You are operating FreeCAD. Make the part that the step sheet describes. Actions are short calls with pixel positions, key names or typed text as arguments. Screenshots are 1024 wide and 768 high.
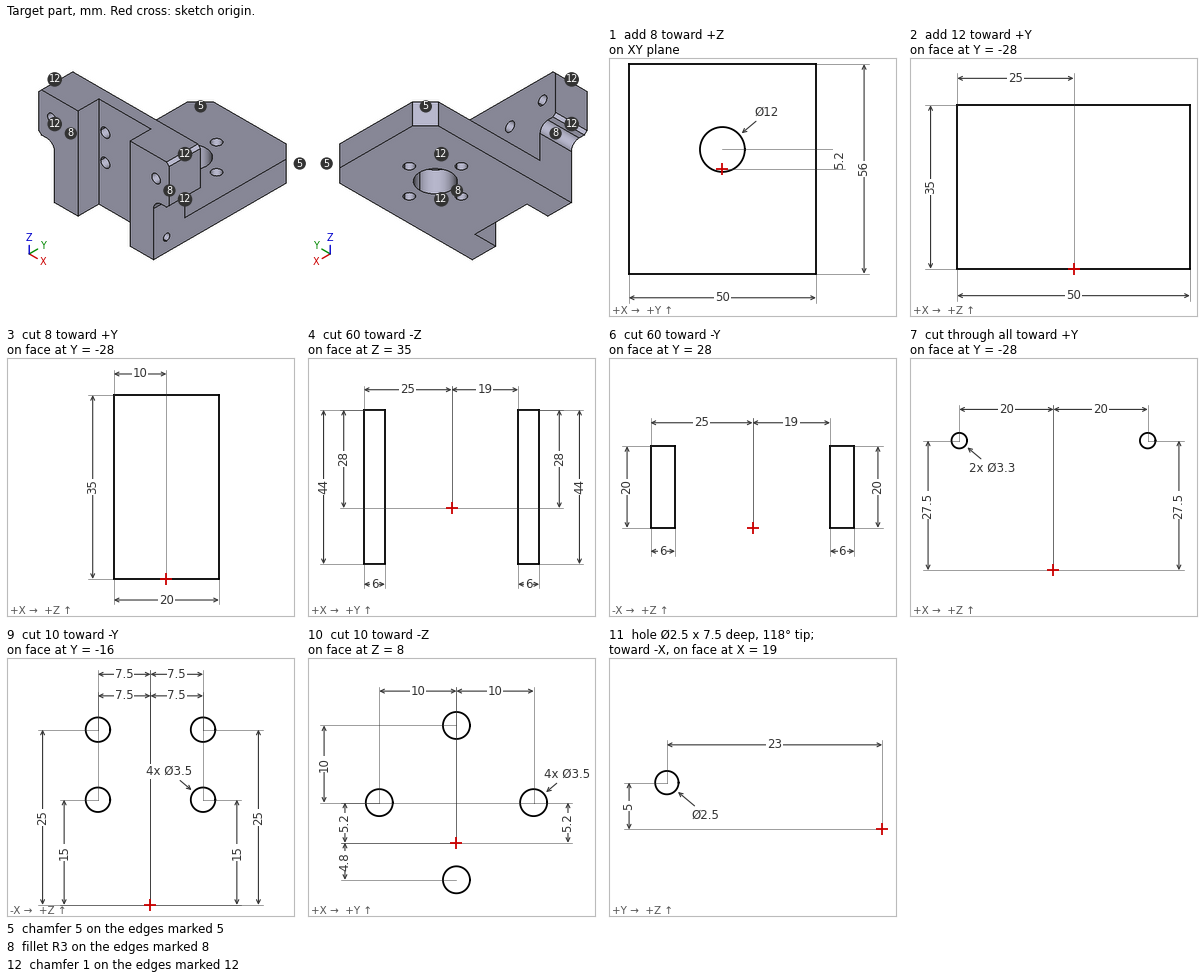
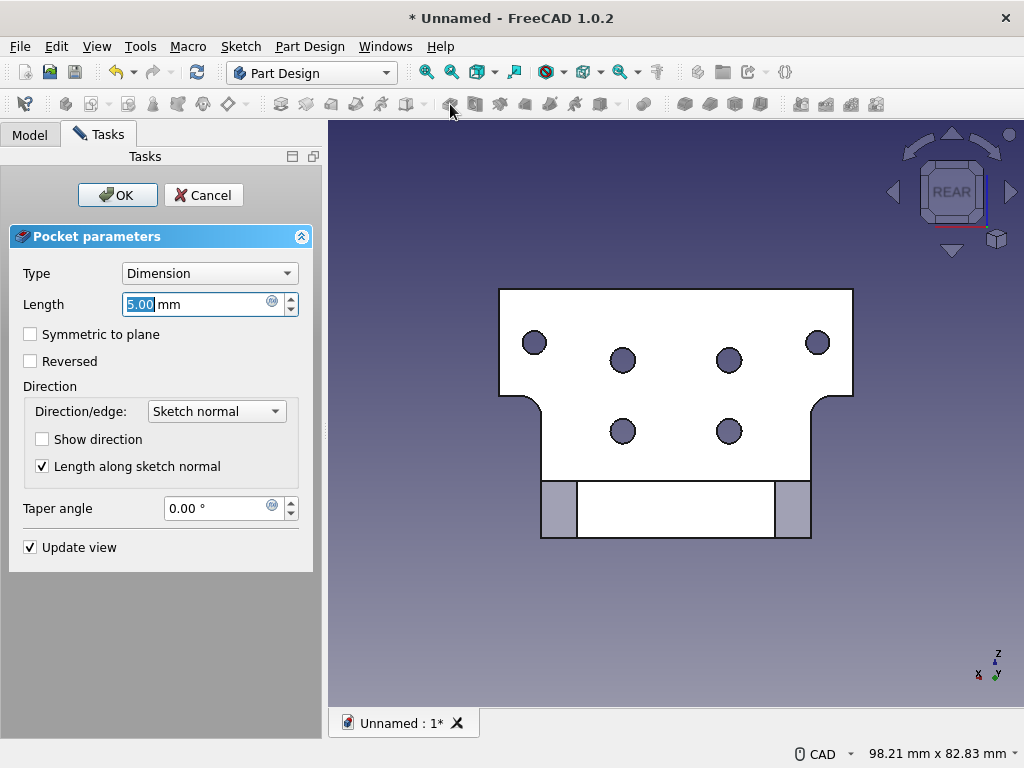
text(10)
key(Tab)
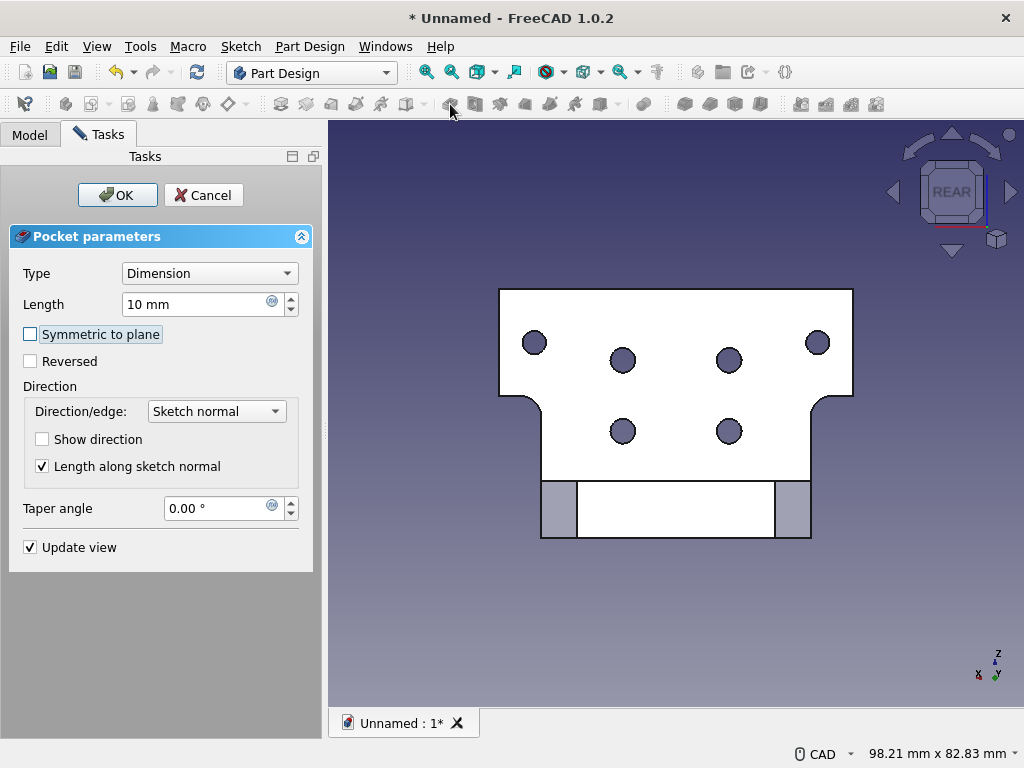
click(118, 195)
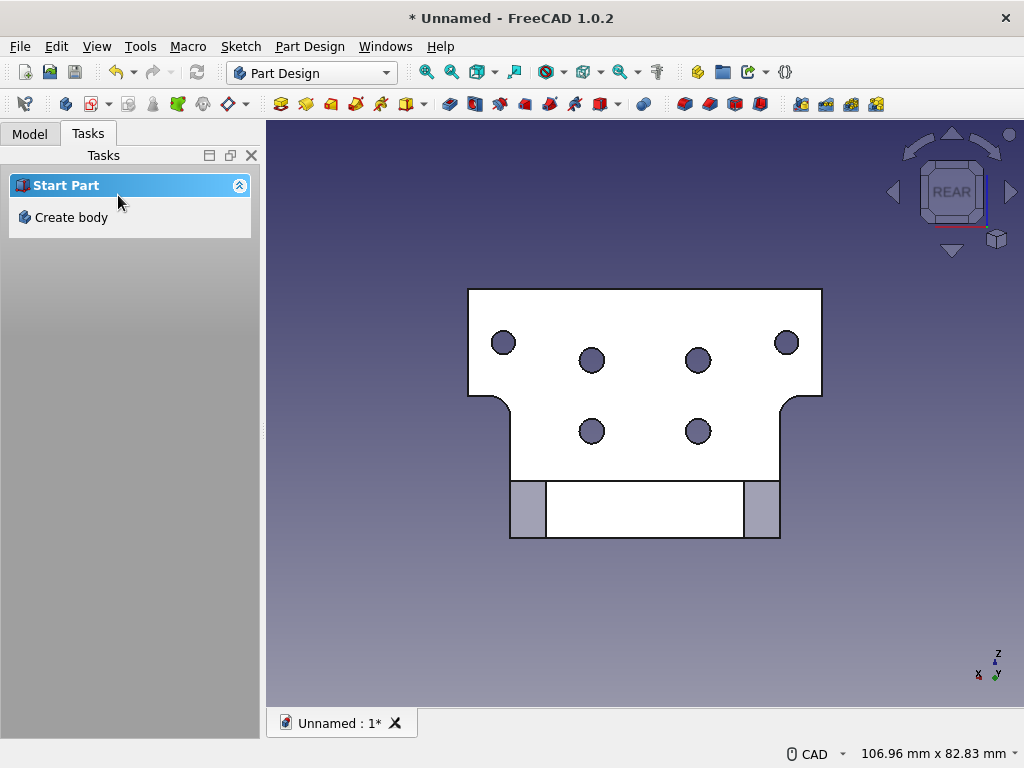
key(0)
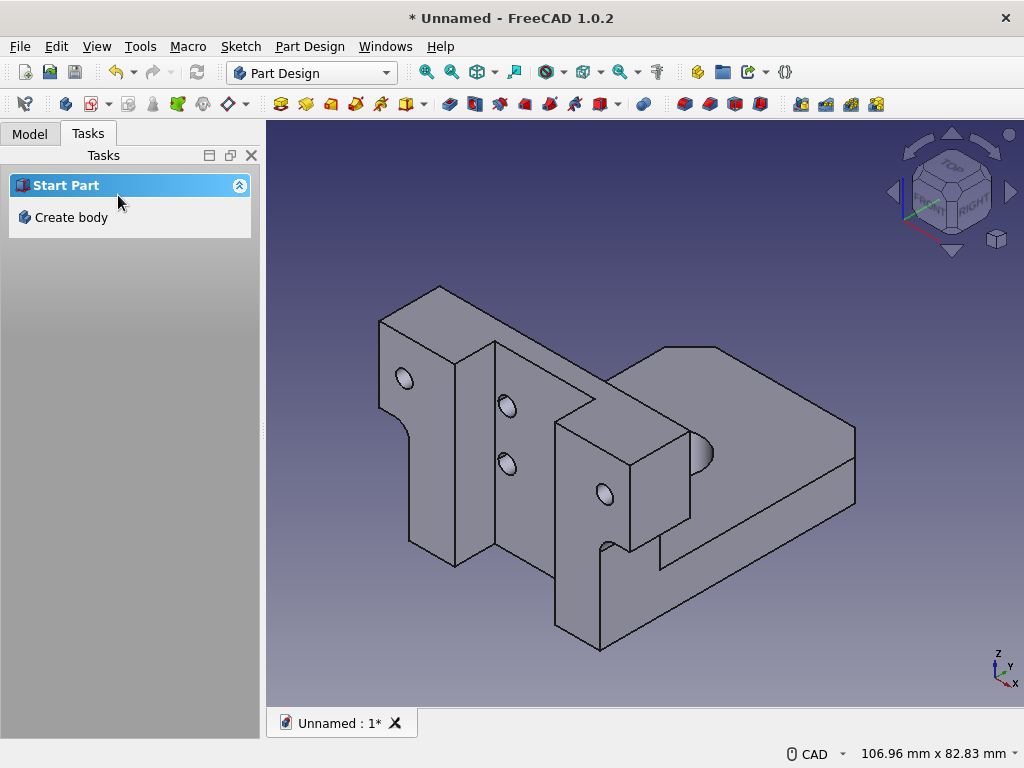
click(711, 398)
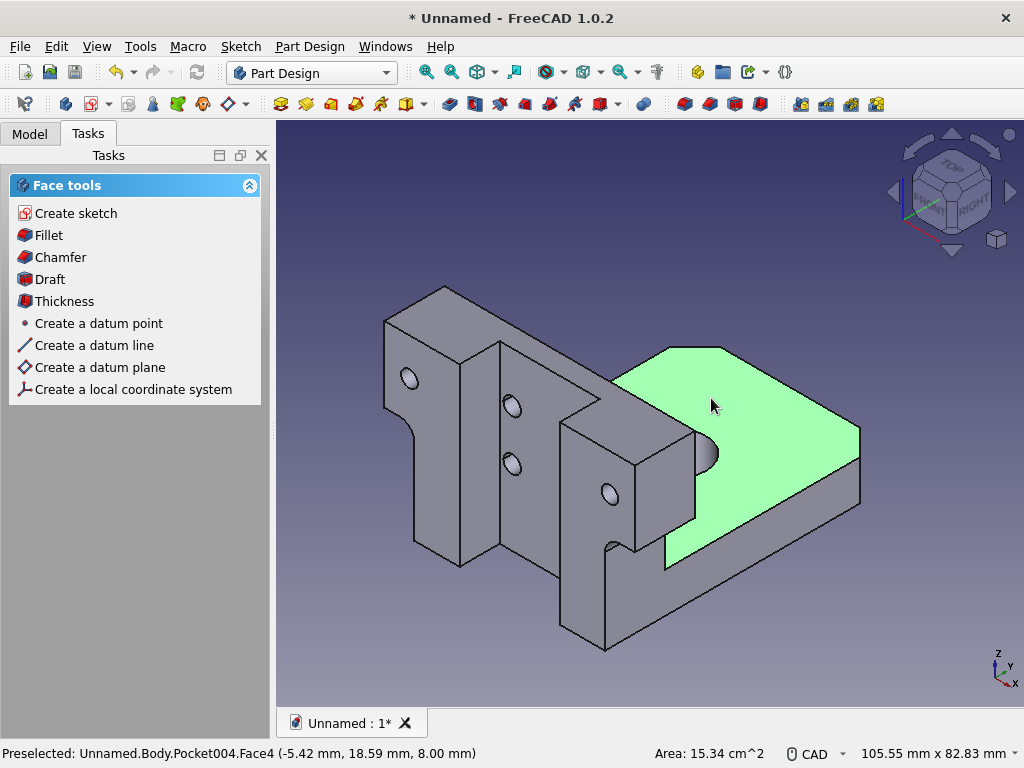
click(90, 104)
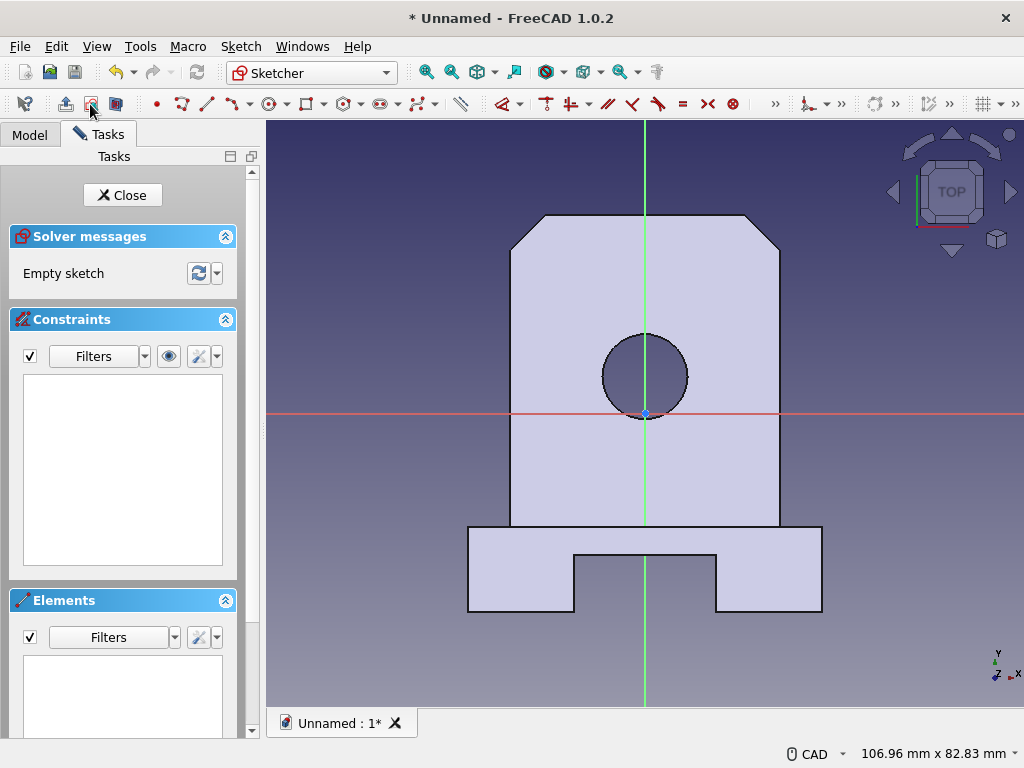
scroll(701, 347, up, 4)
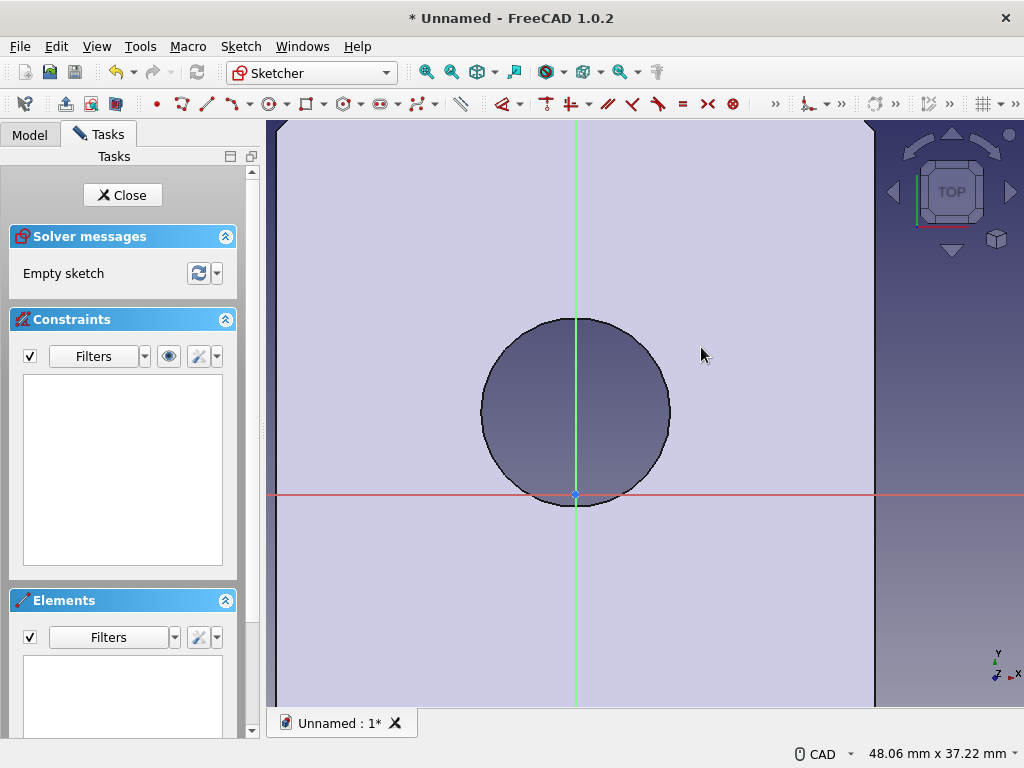
click(268, 104)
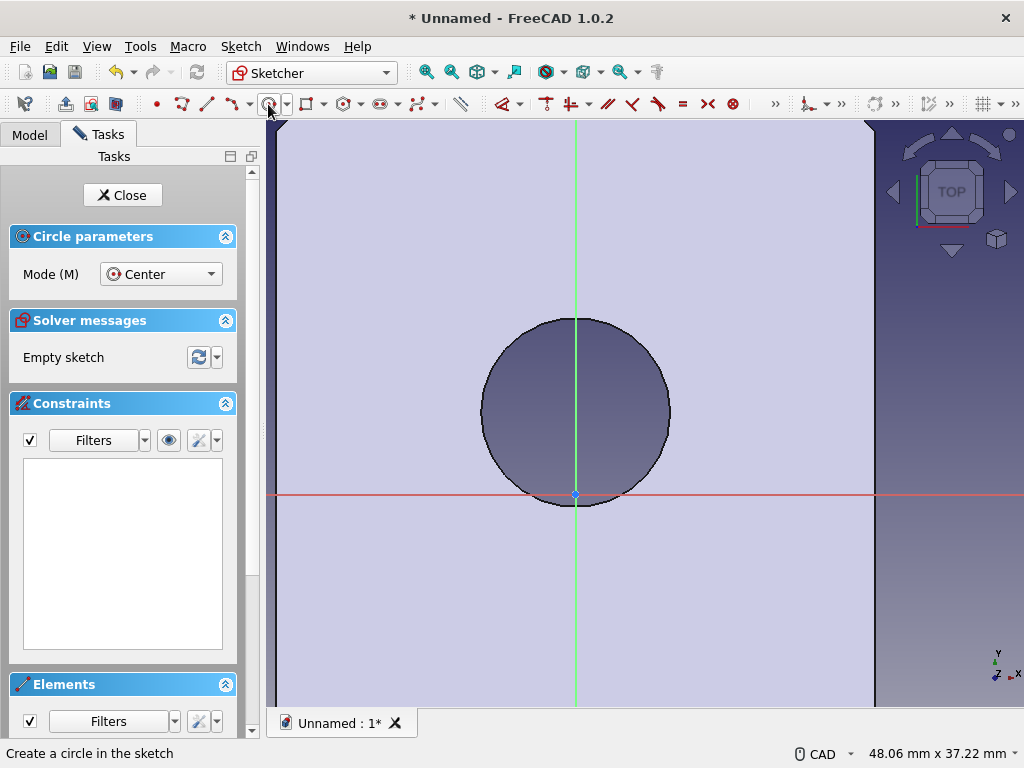
click(733, 413)
move(753, 393)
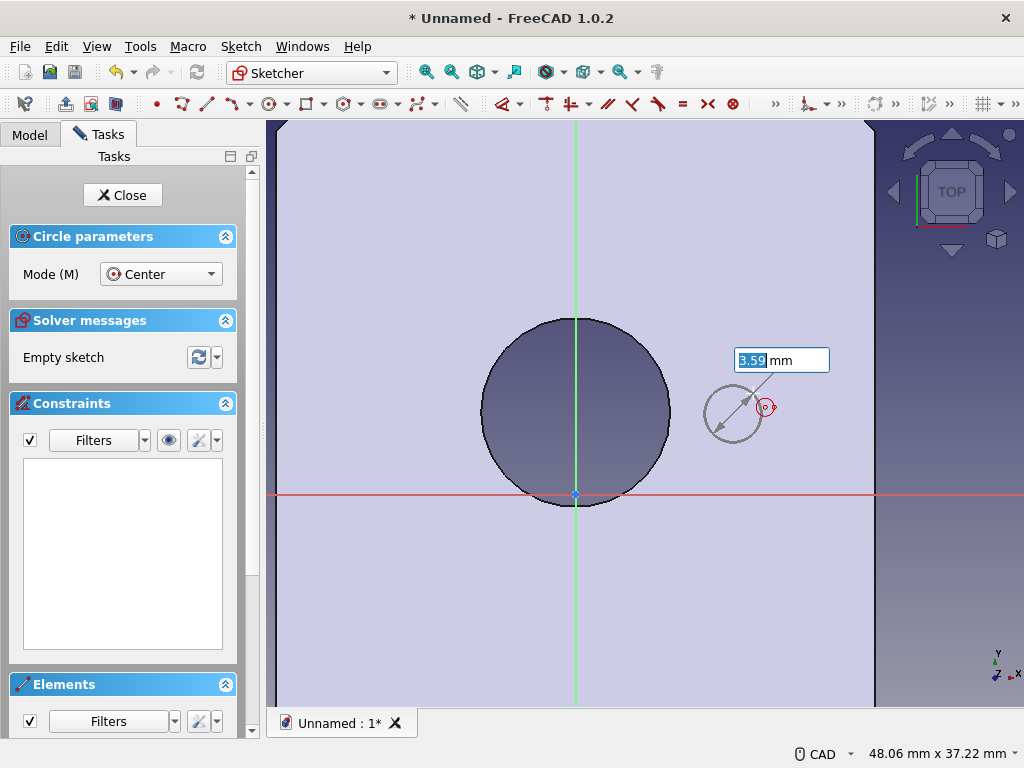
text(3.5)
key(Return)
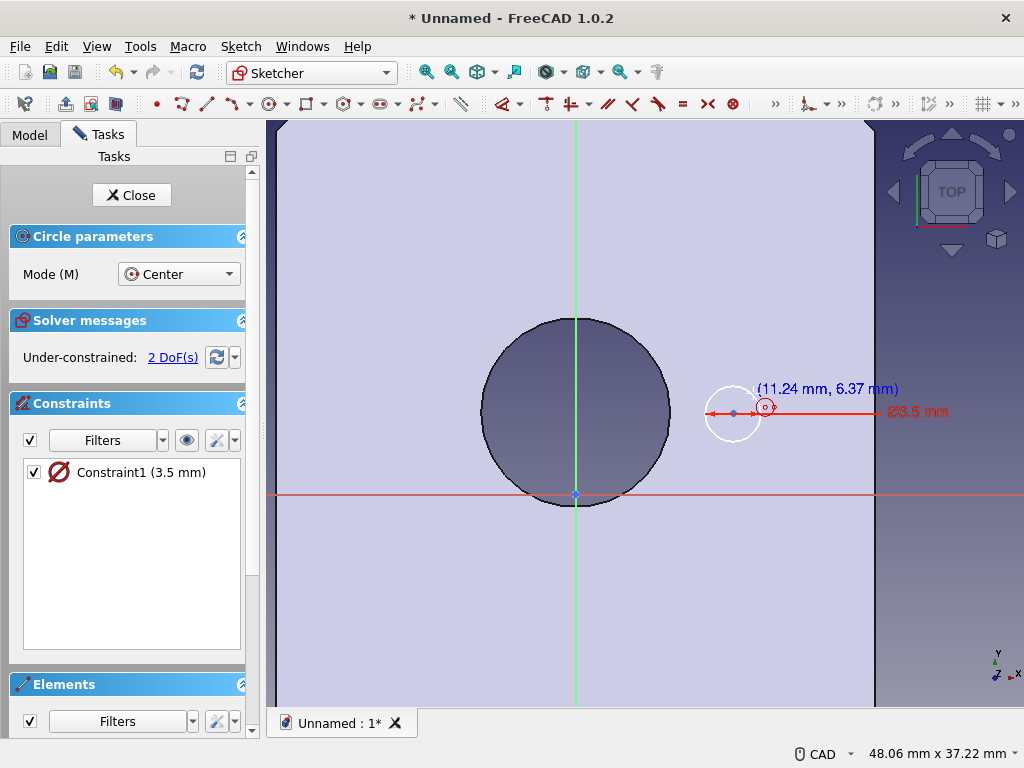
click(576, 255)
move(595, 235)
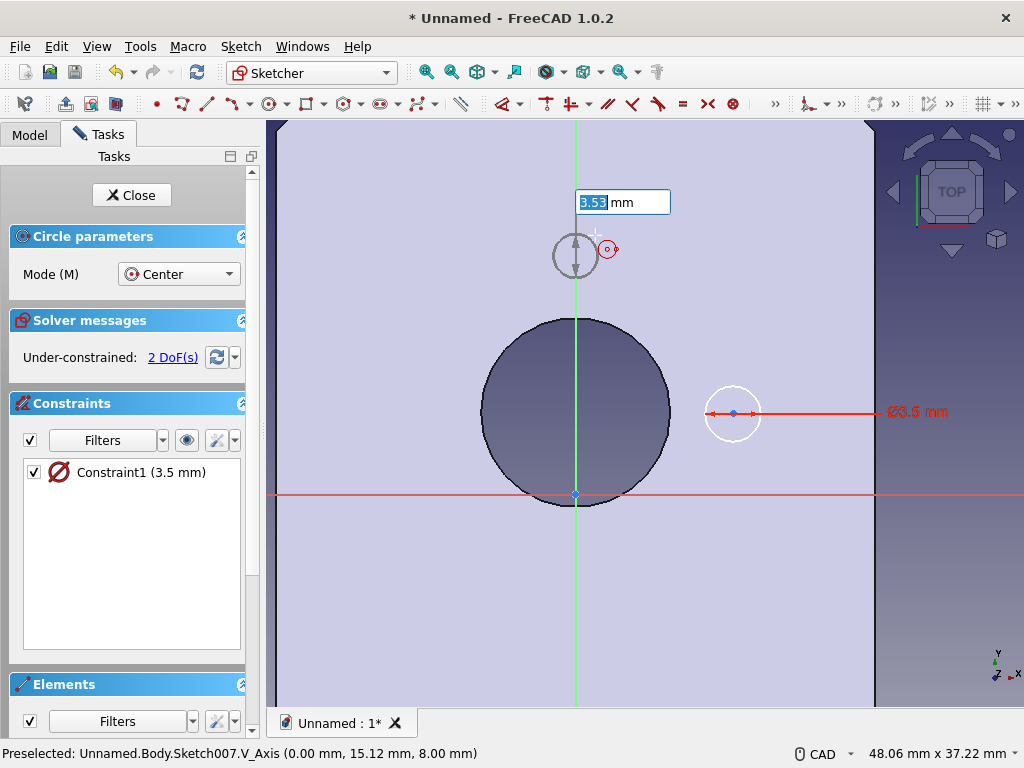
text(3.5)
key(Return)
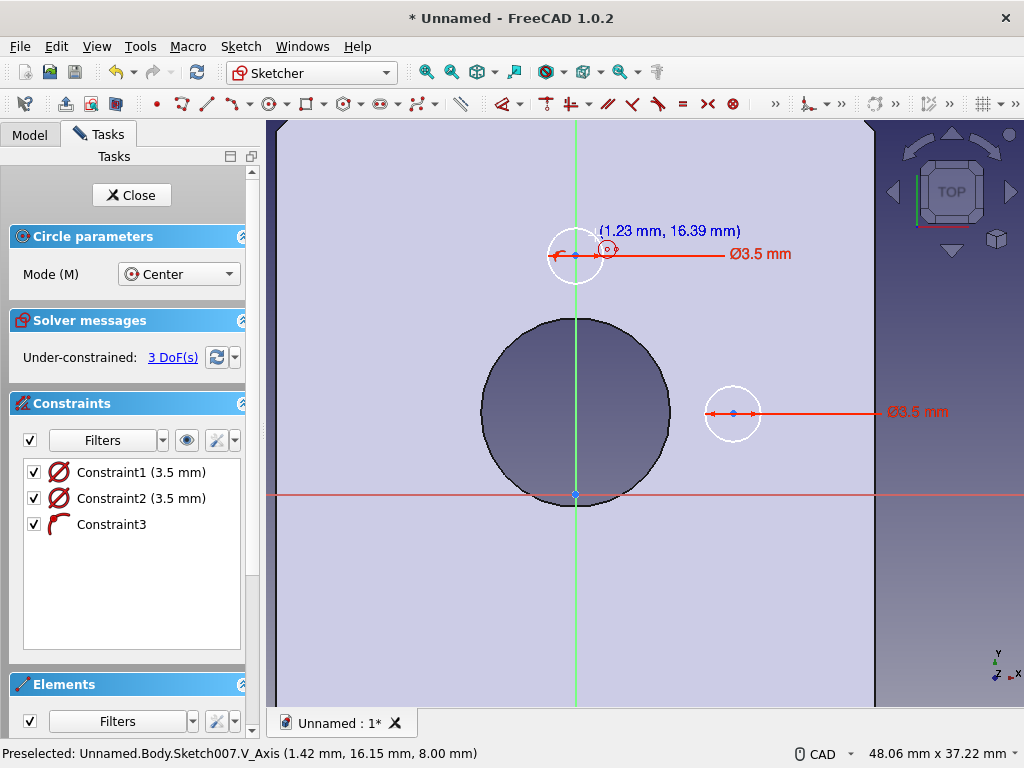
click(418, 413)
move(437, 393)